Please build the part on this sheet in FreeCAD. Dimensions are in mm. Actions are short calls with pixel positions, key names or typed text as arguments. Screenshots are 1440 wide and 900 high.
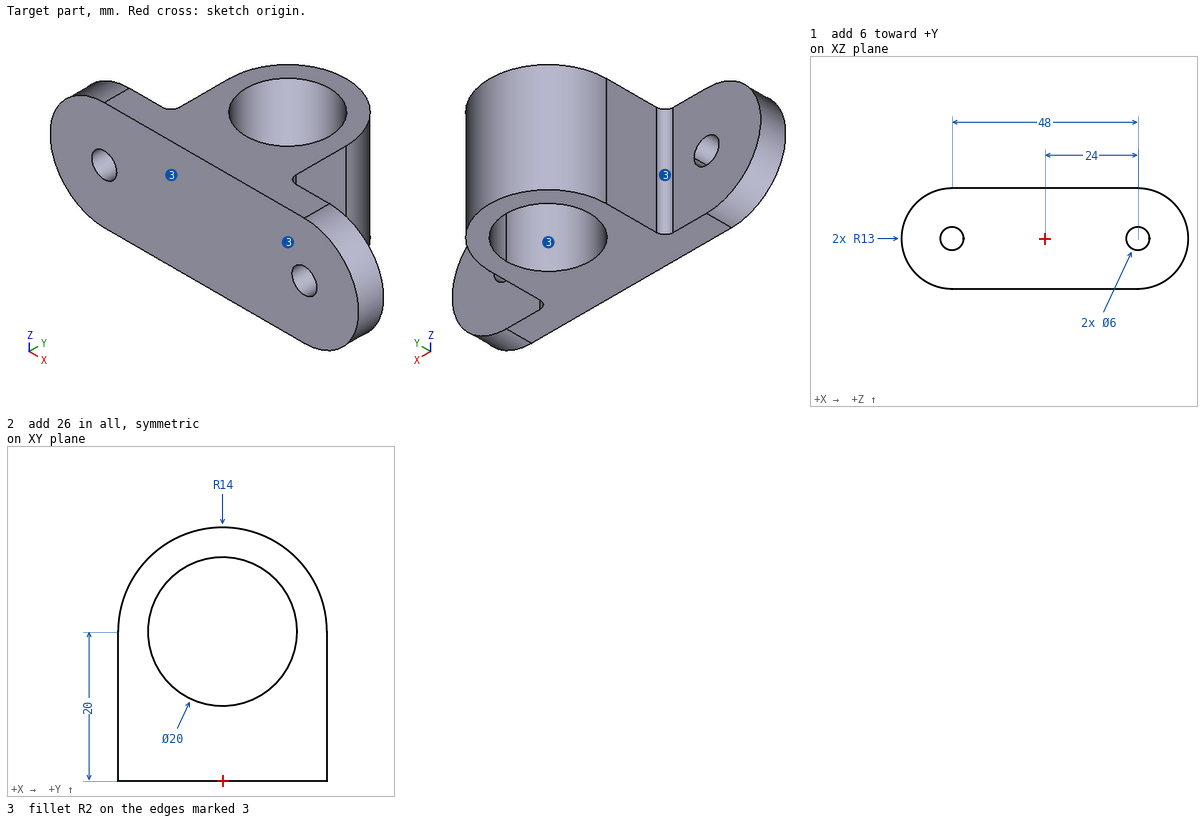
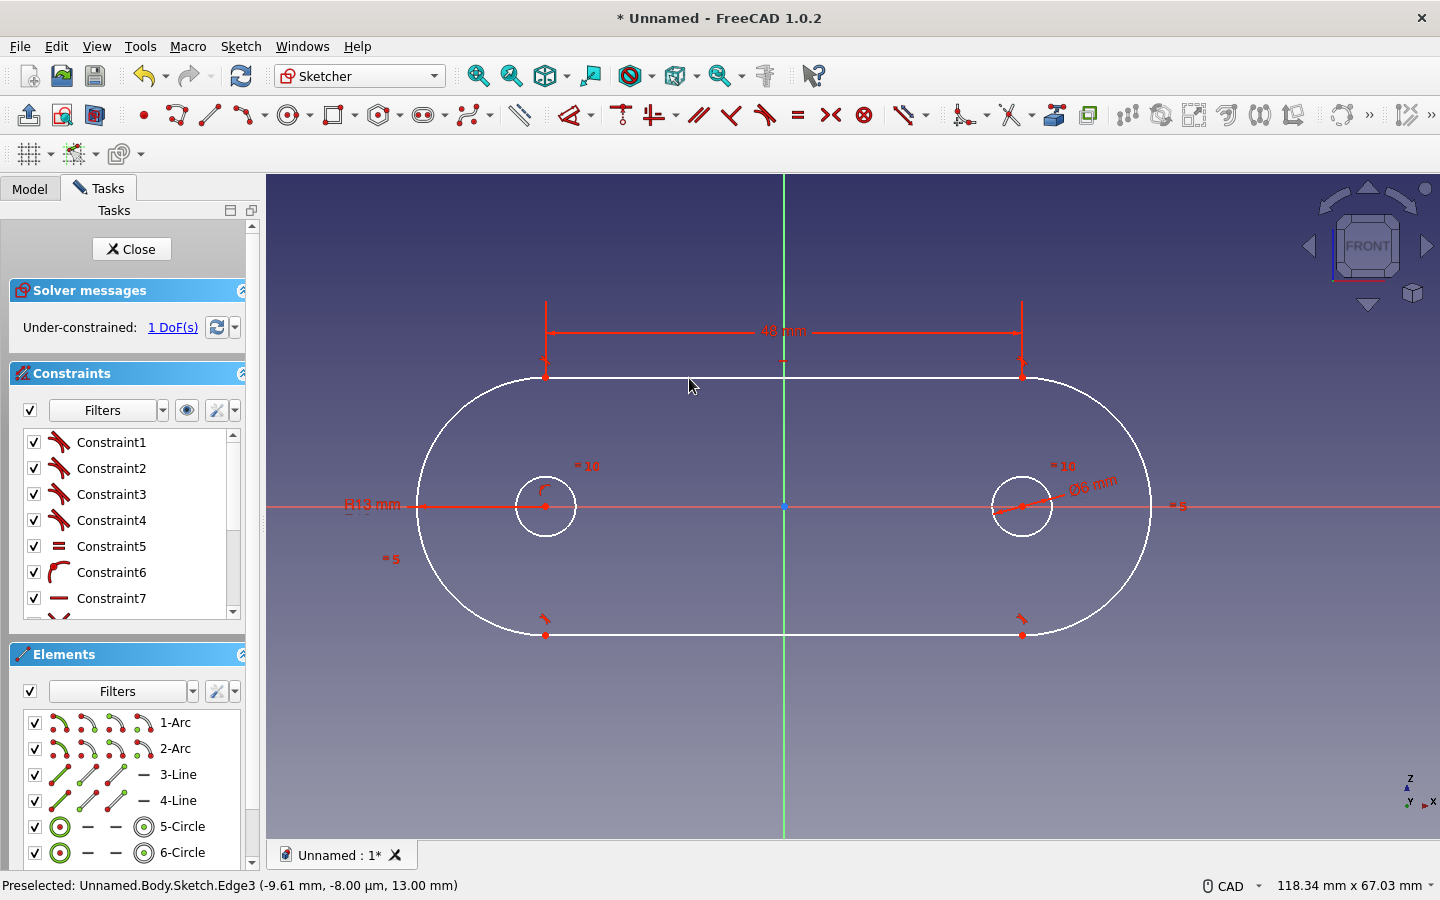
click(1022, 506)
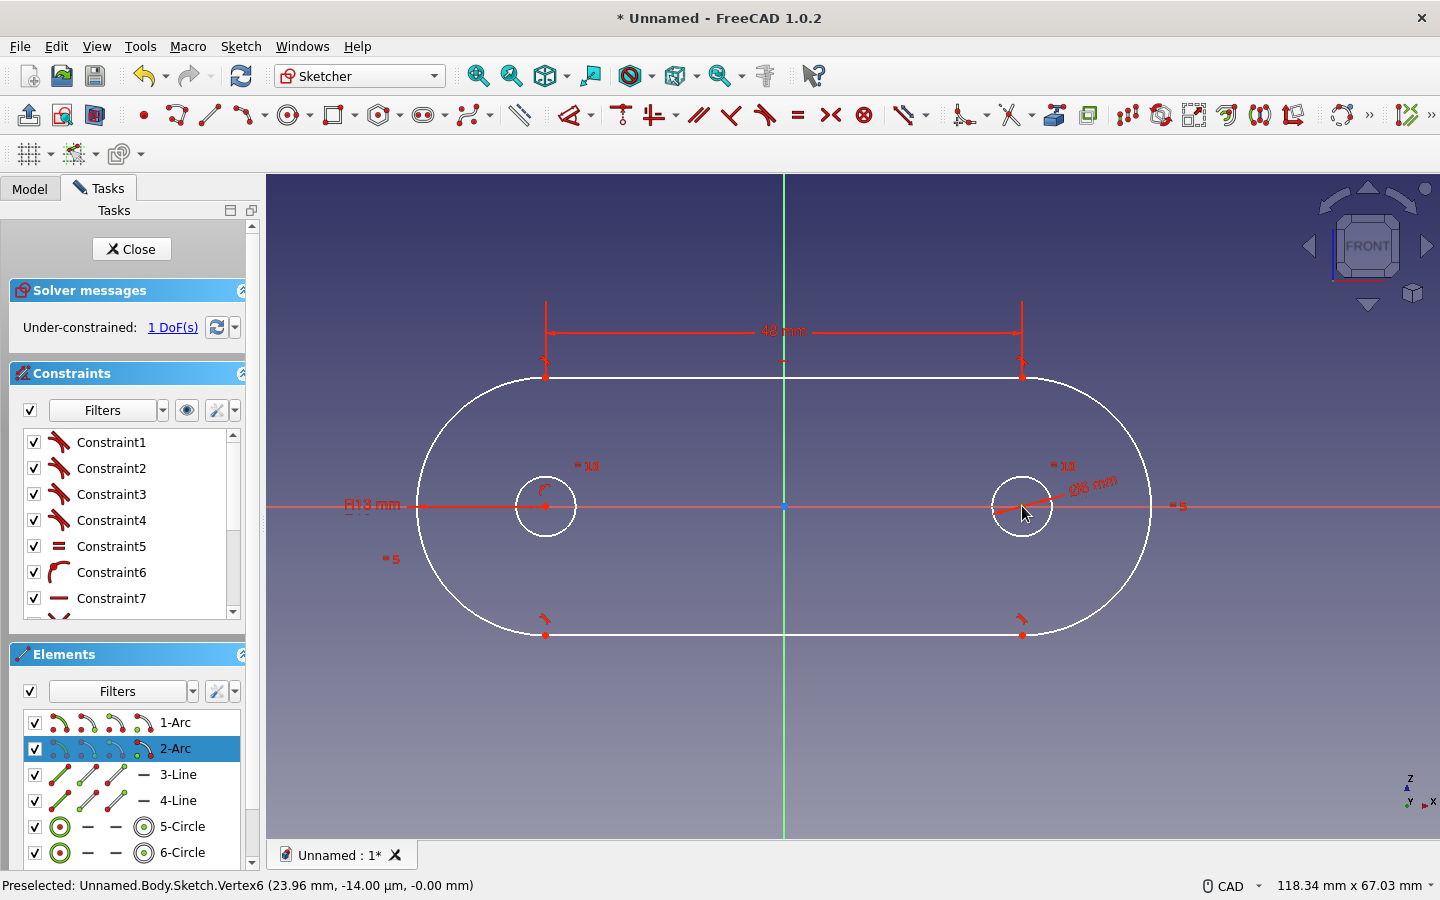
key(l)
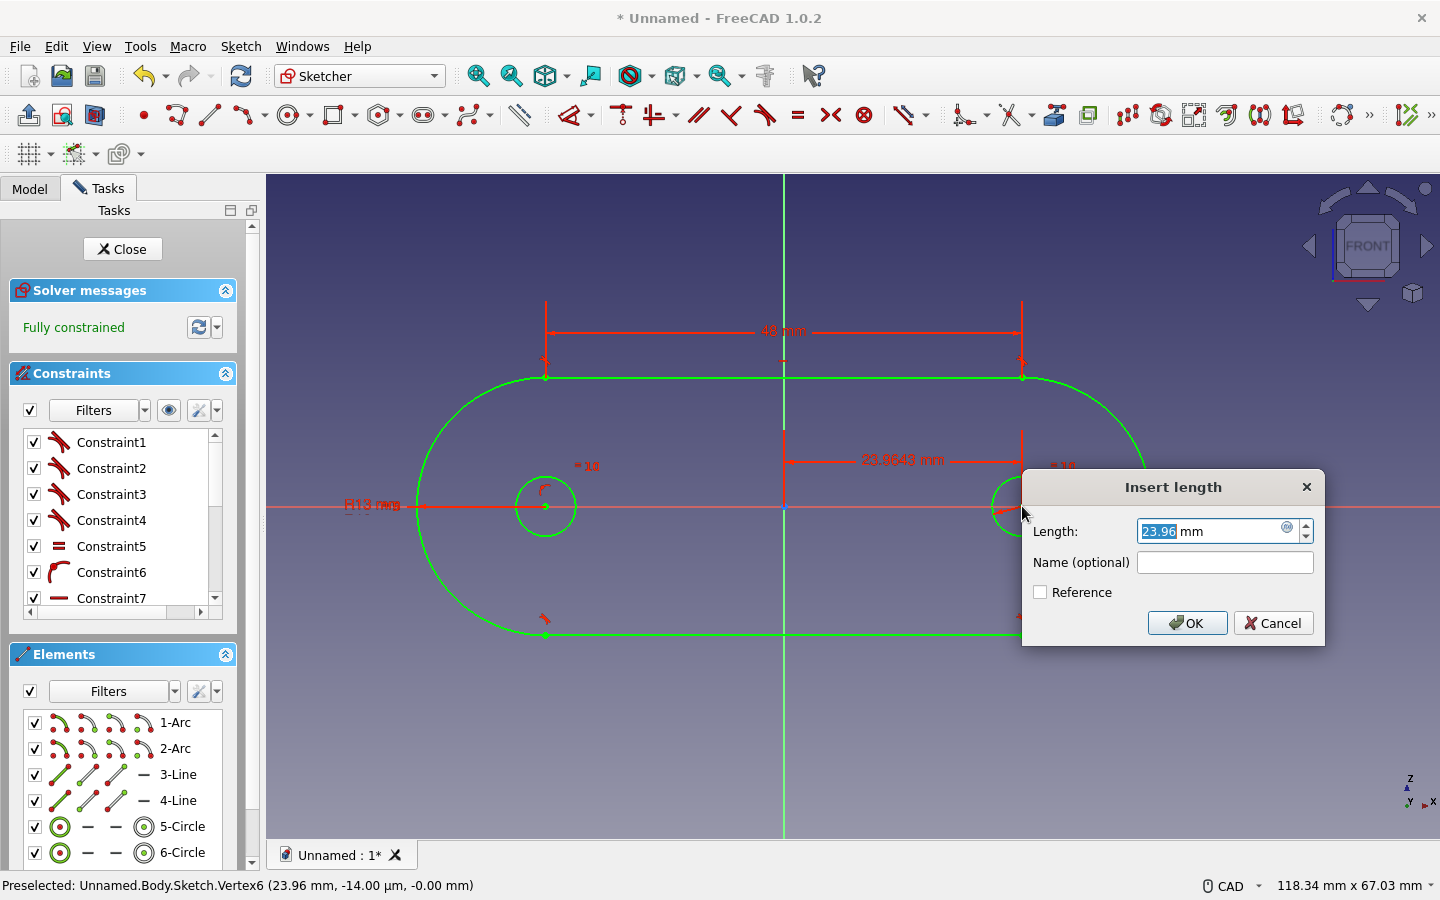
text(24)
key(Return)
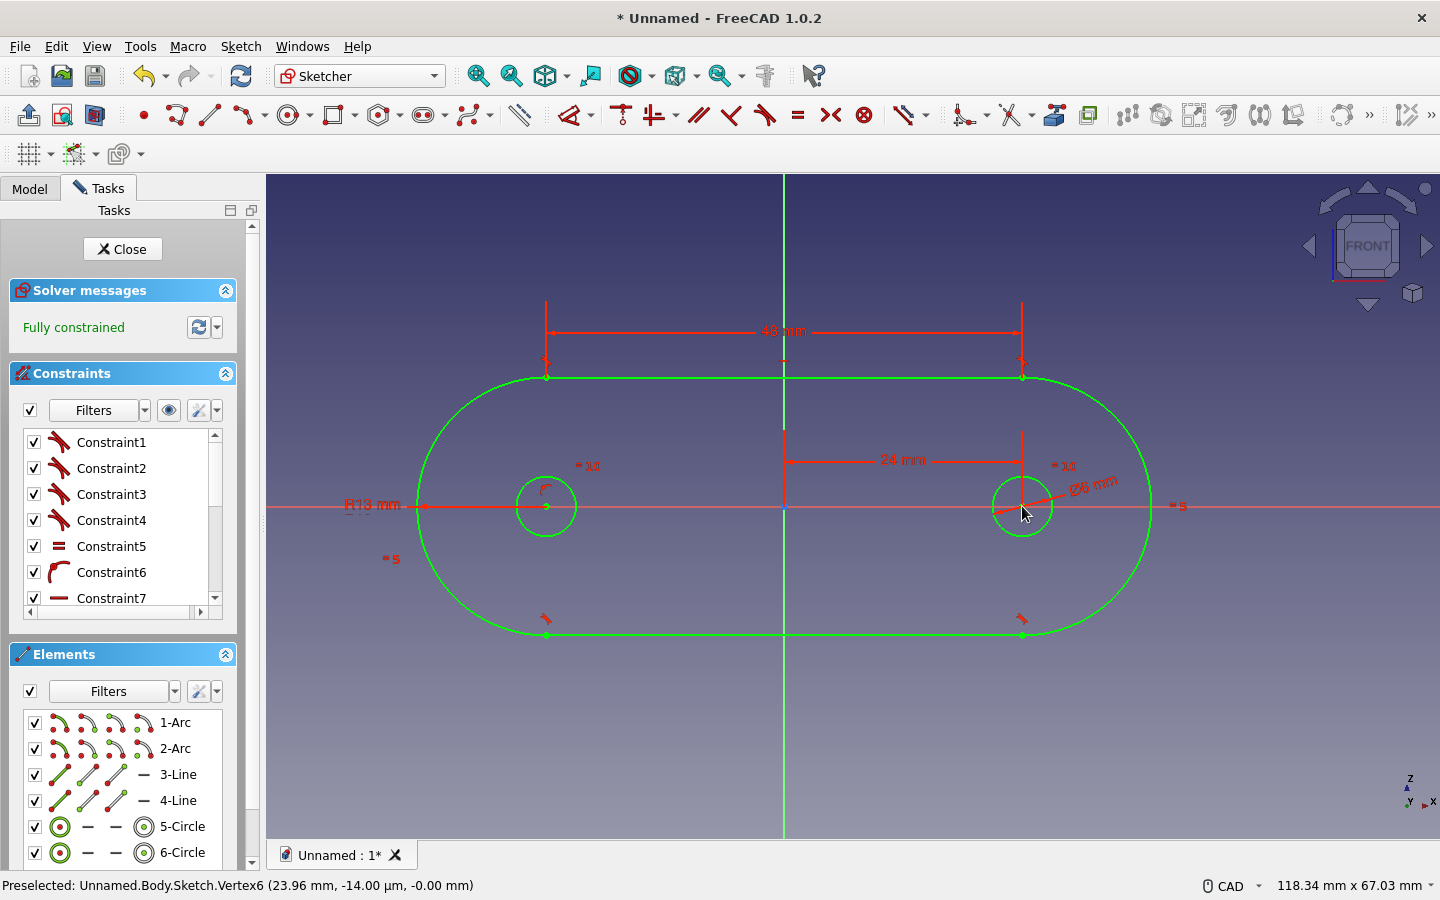
click(123, 249)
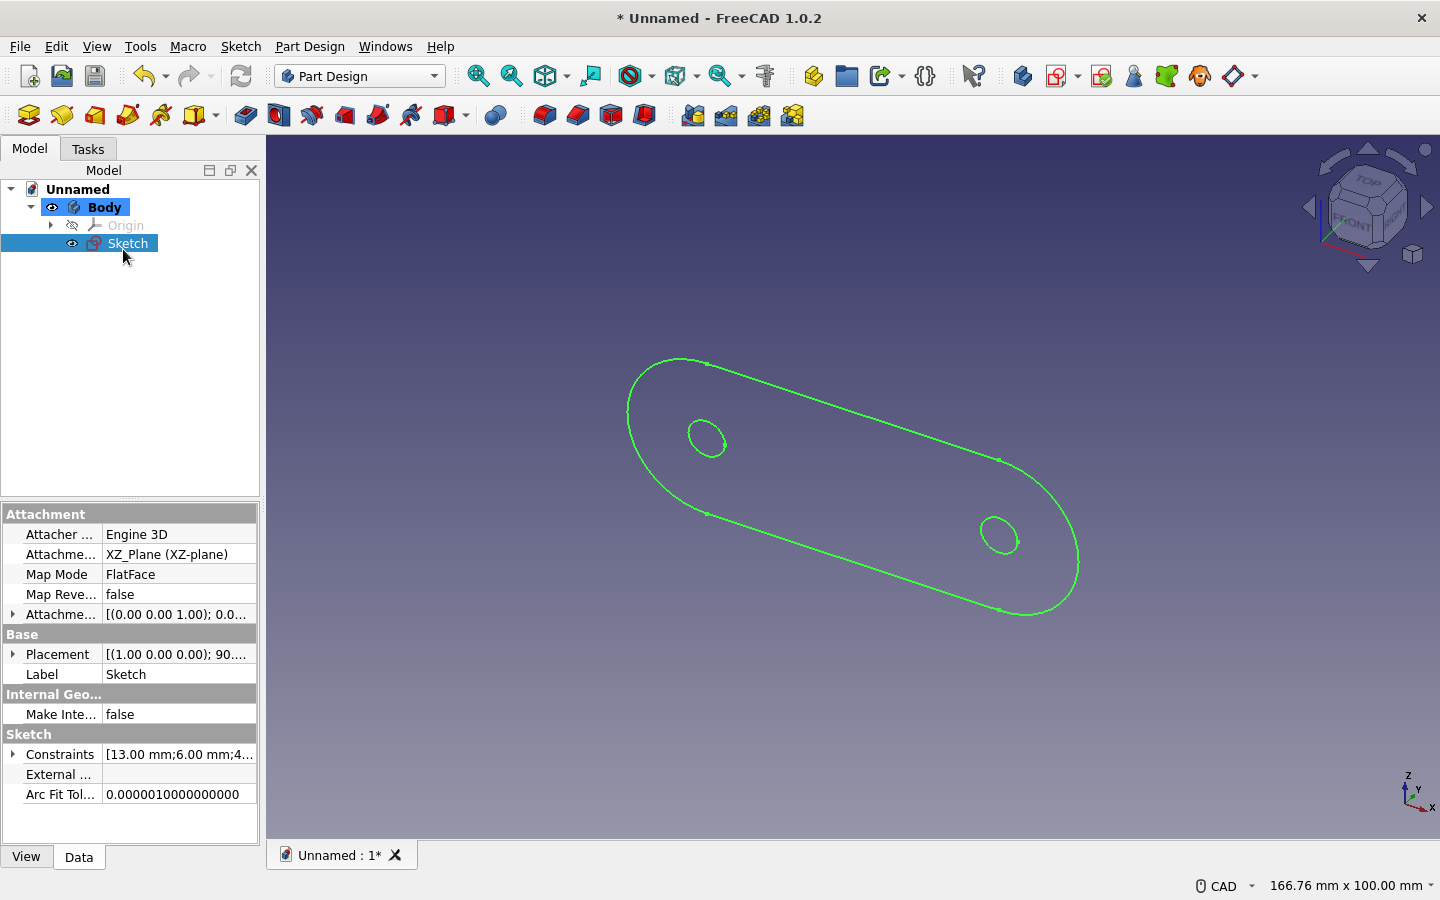
click(29, 116)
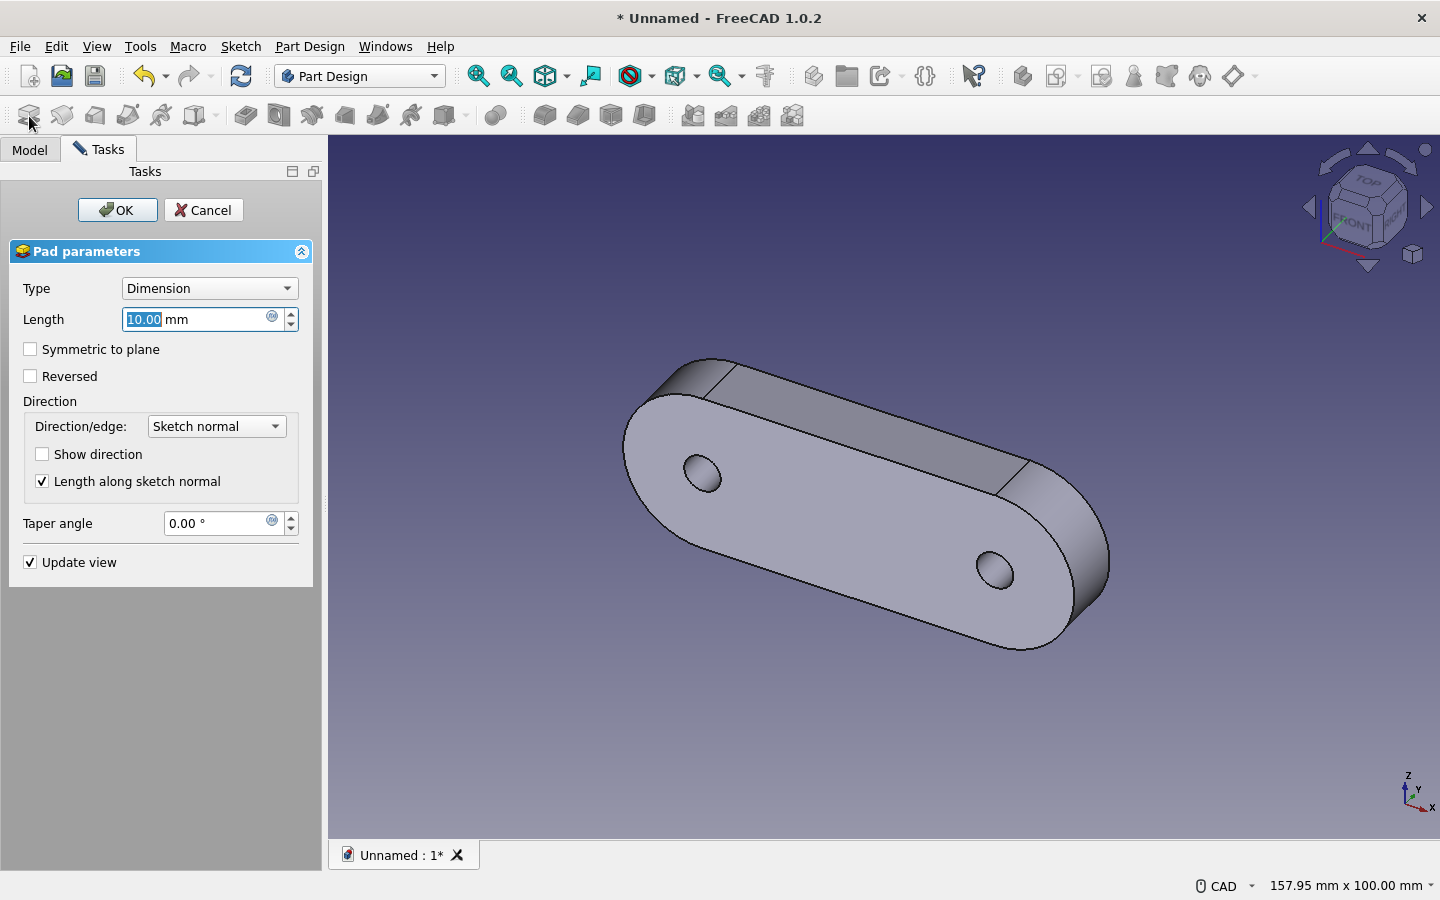
text(6)
key(Tab)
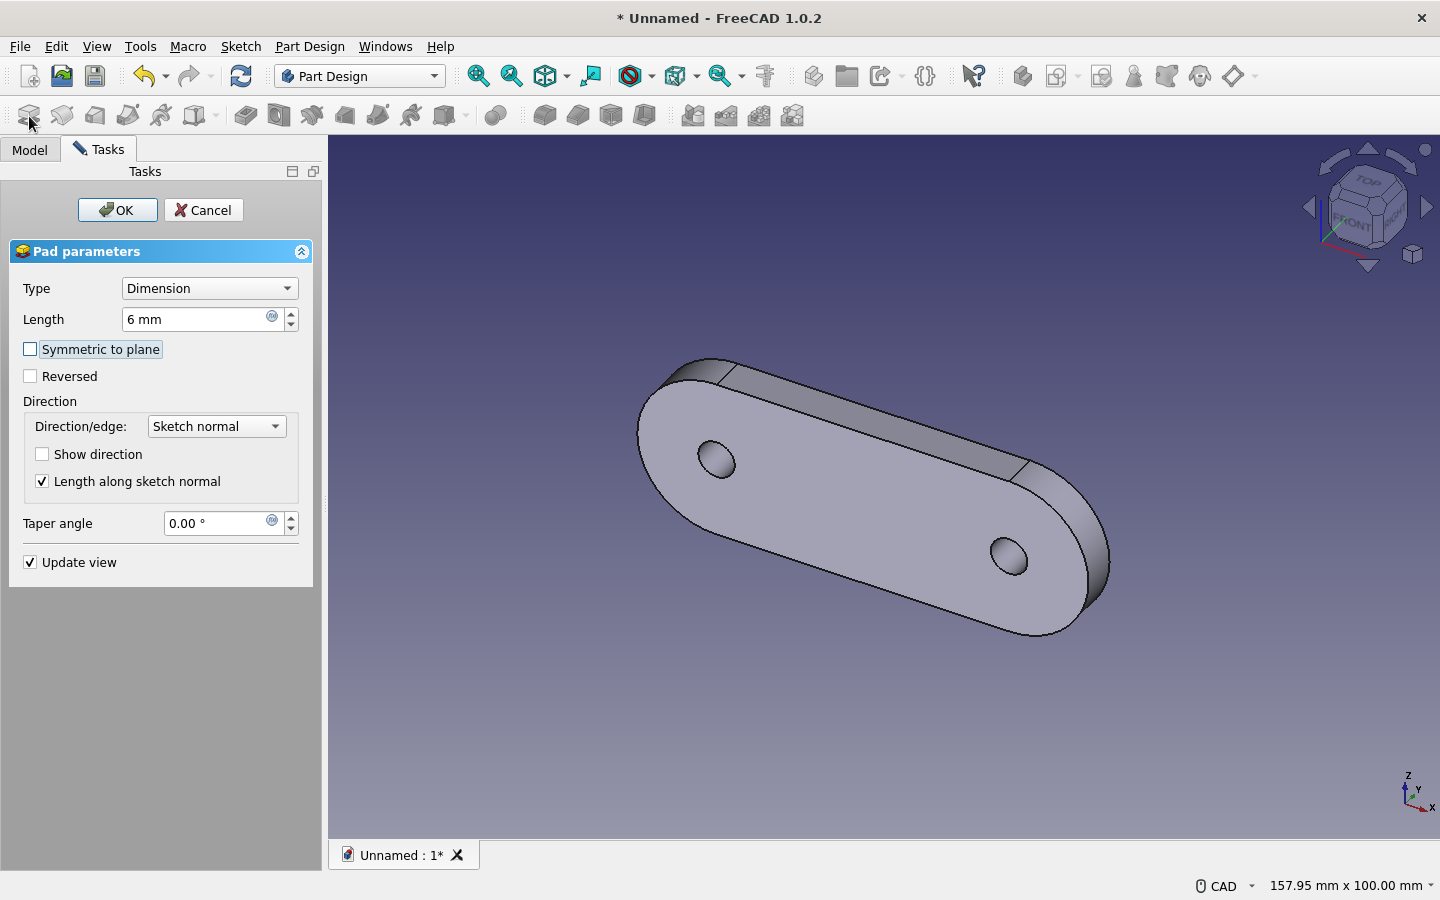
click(31, 376)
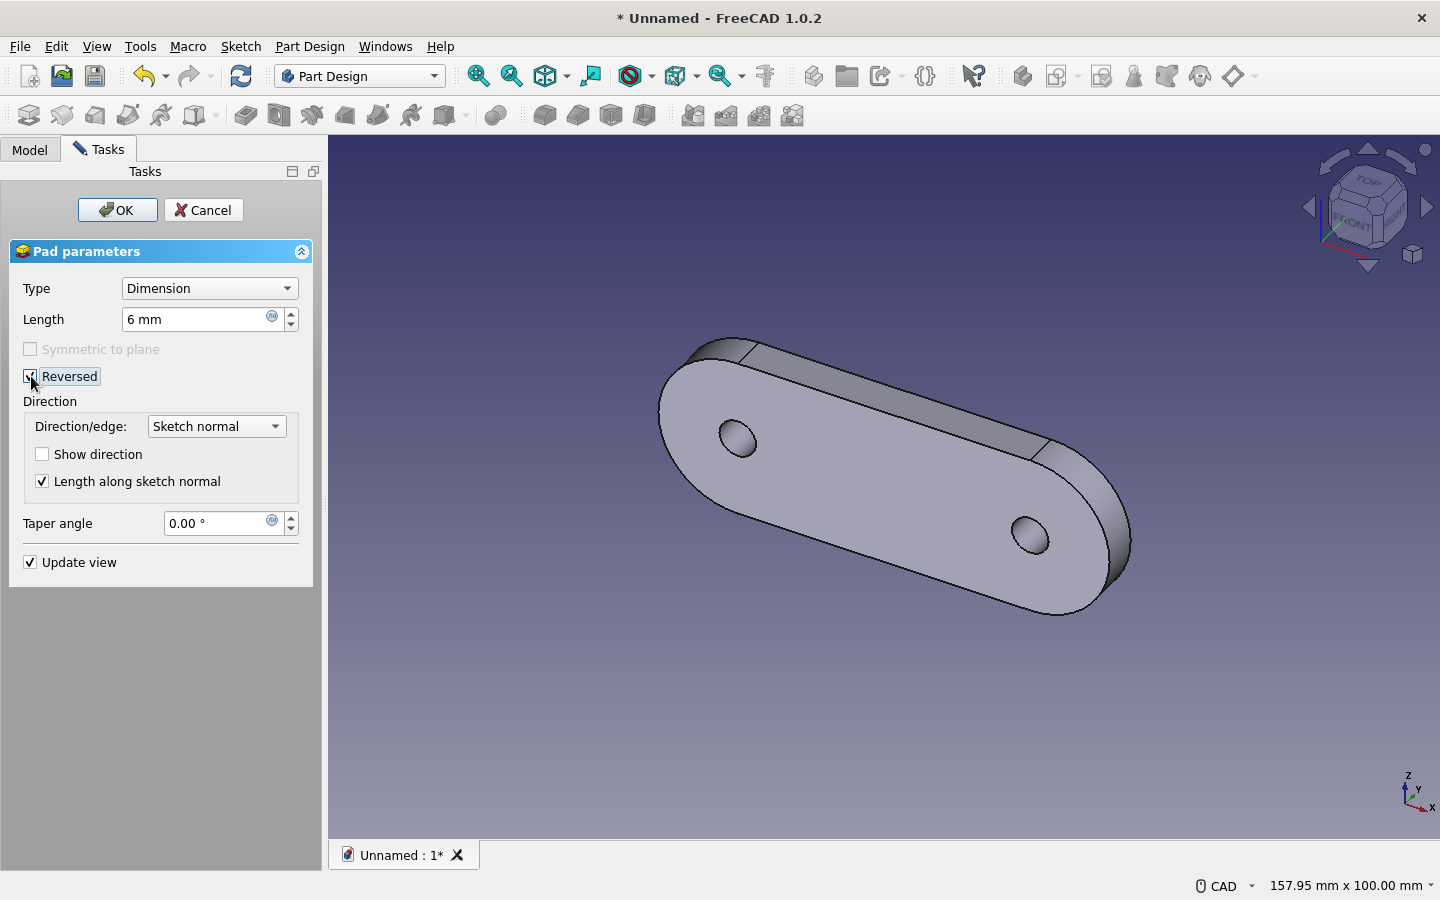
click(118, 210)